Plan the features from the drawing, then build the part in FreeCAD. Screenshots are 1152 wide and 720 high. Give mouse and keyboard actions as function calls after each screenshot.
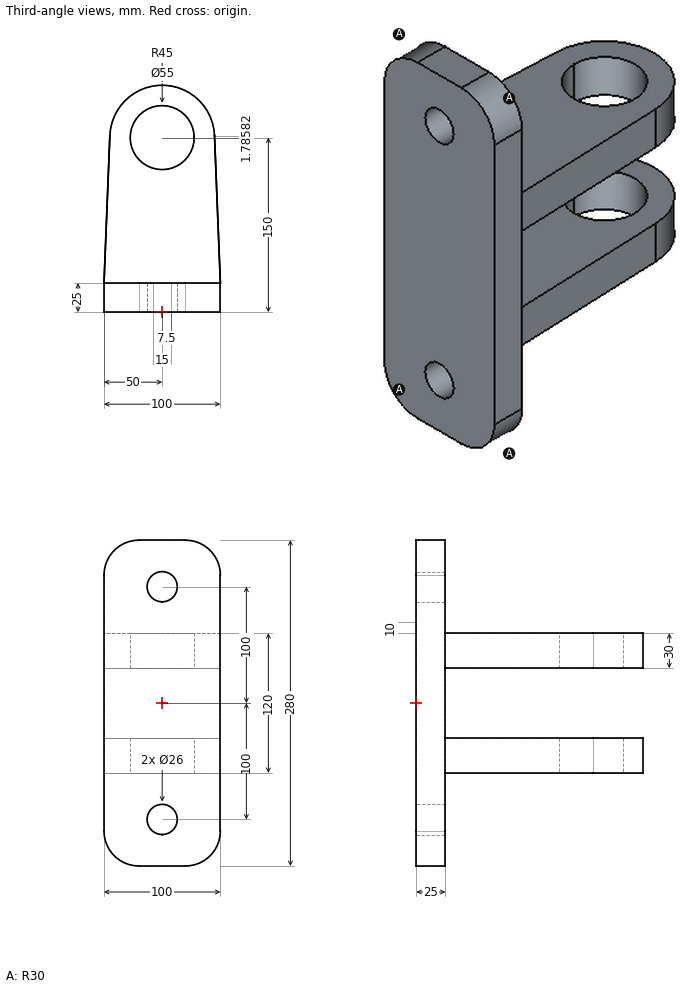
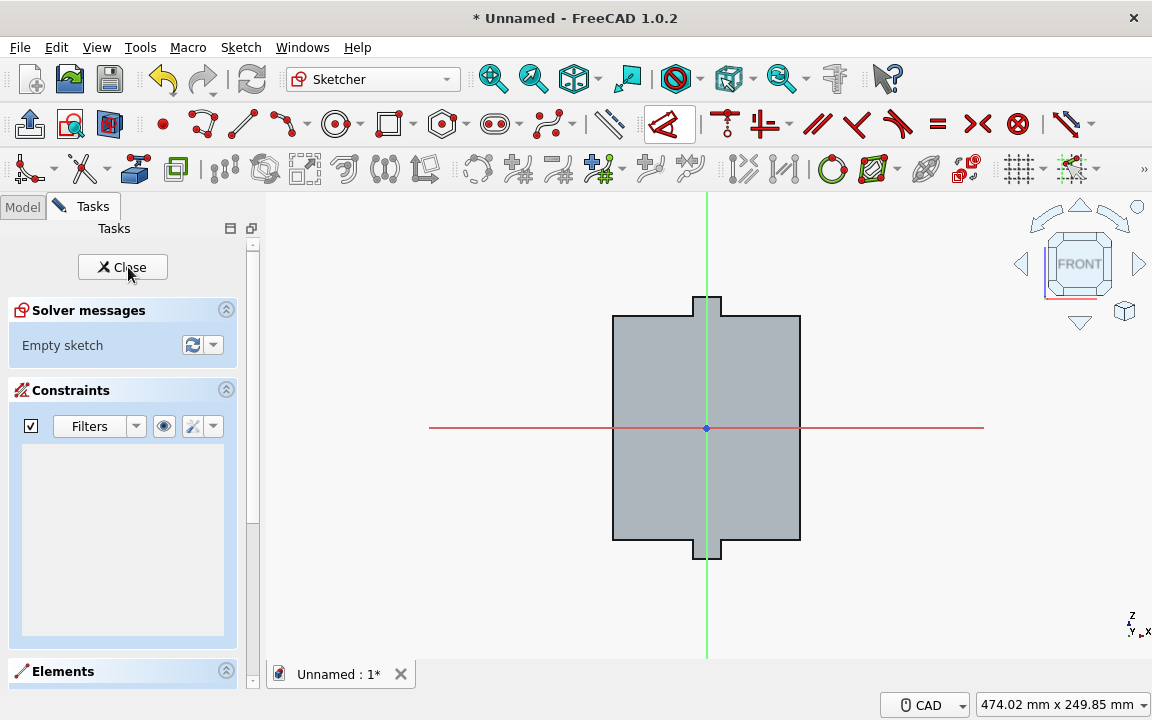
scroll(560, 422, down, 3)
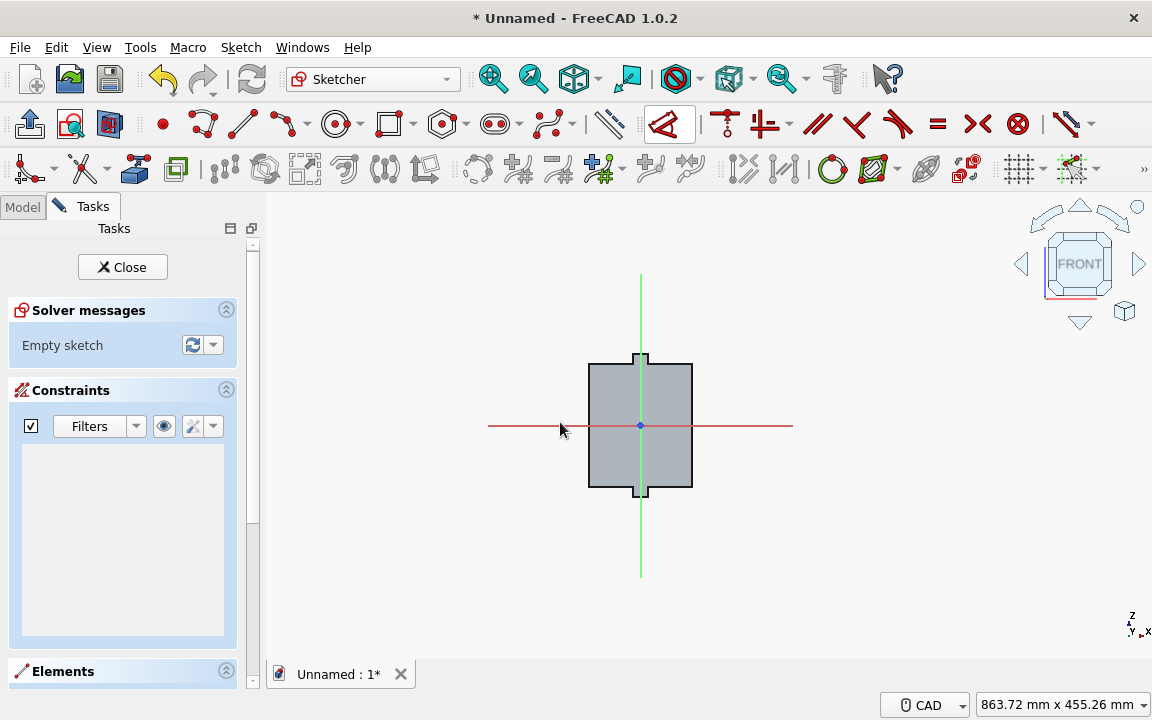
key(g)
key(v)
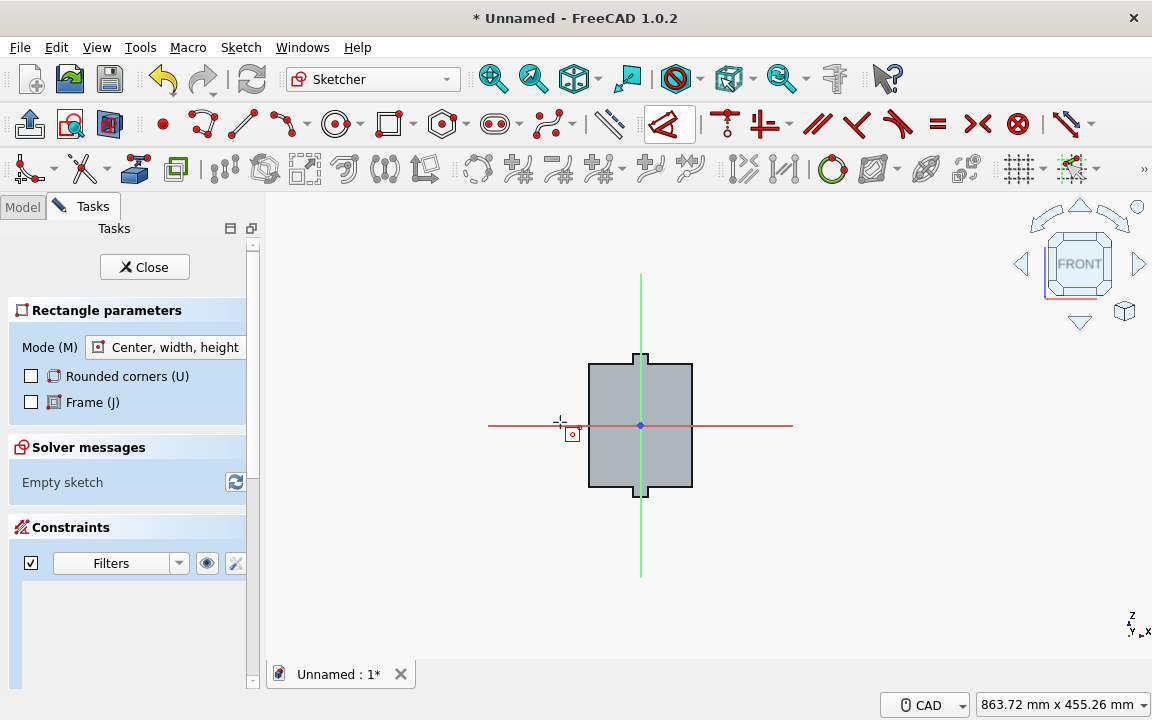
click(641, 426)
click(692, 282)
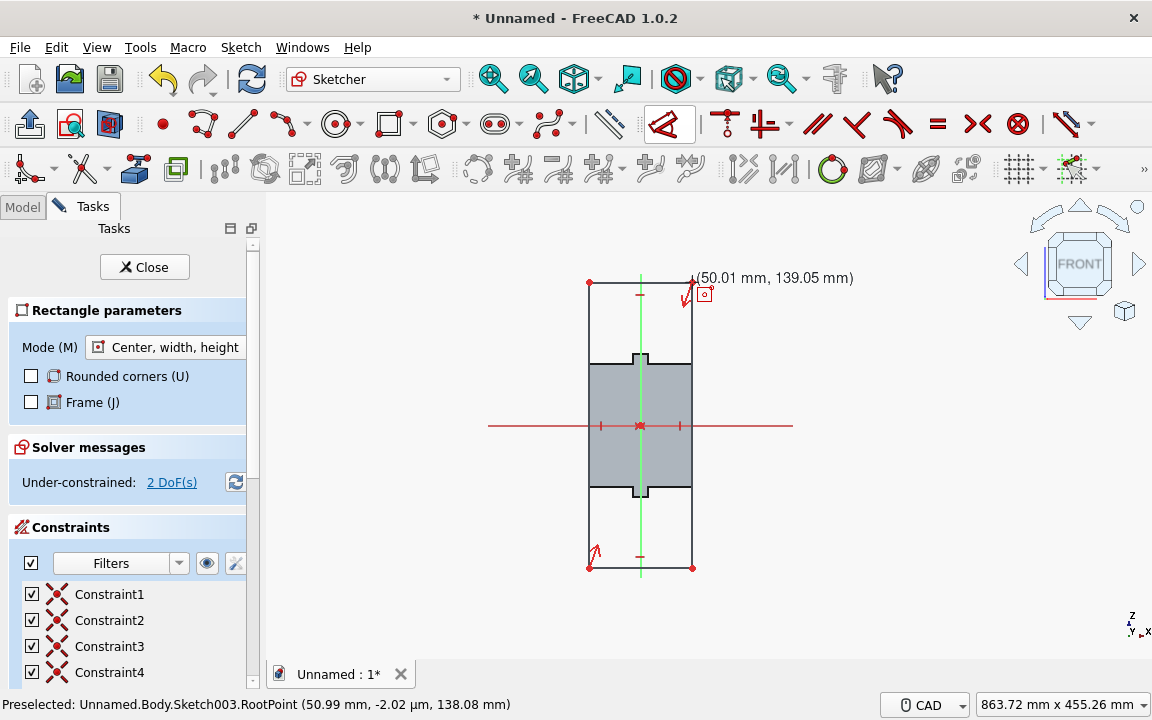
click(336, 124)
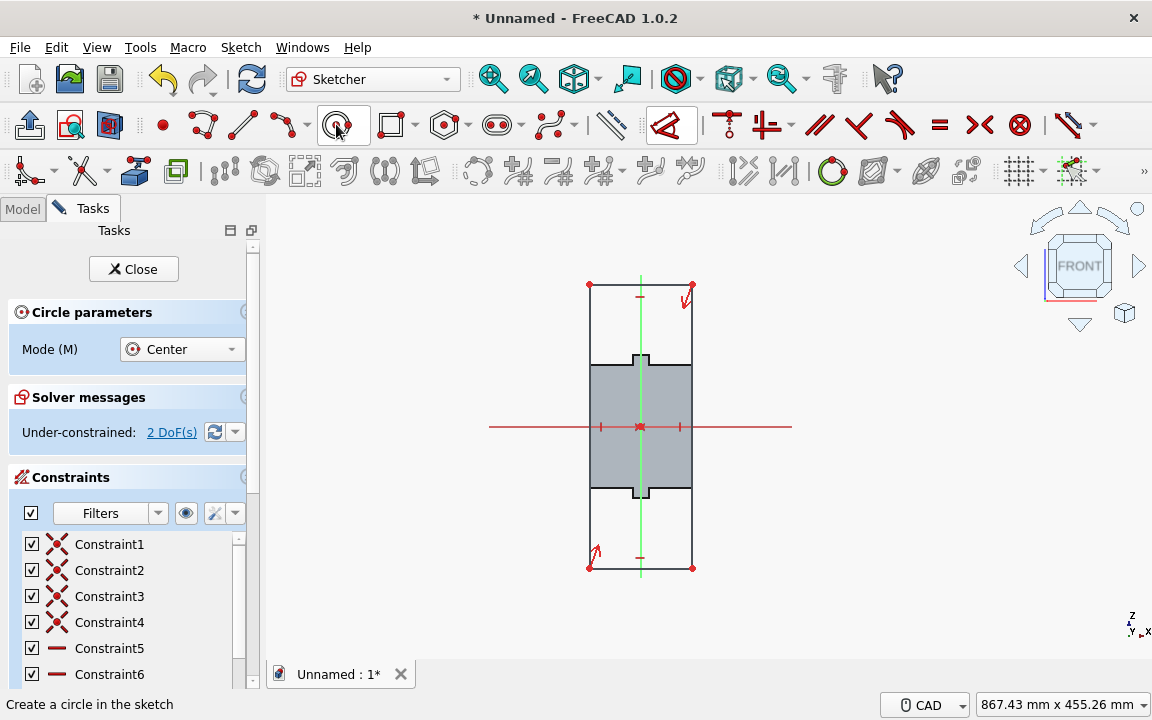
scroll(641, 529, up, 3)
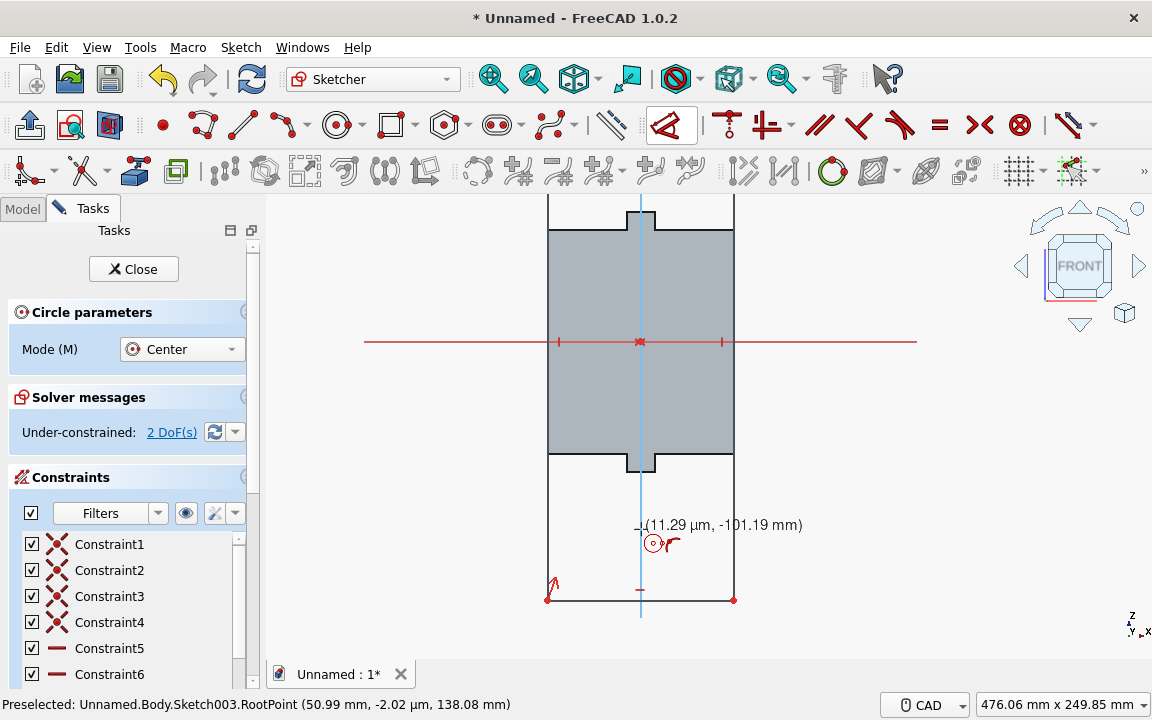
click(641, 528)
click(658, 511)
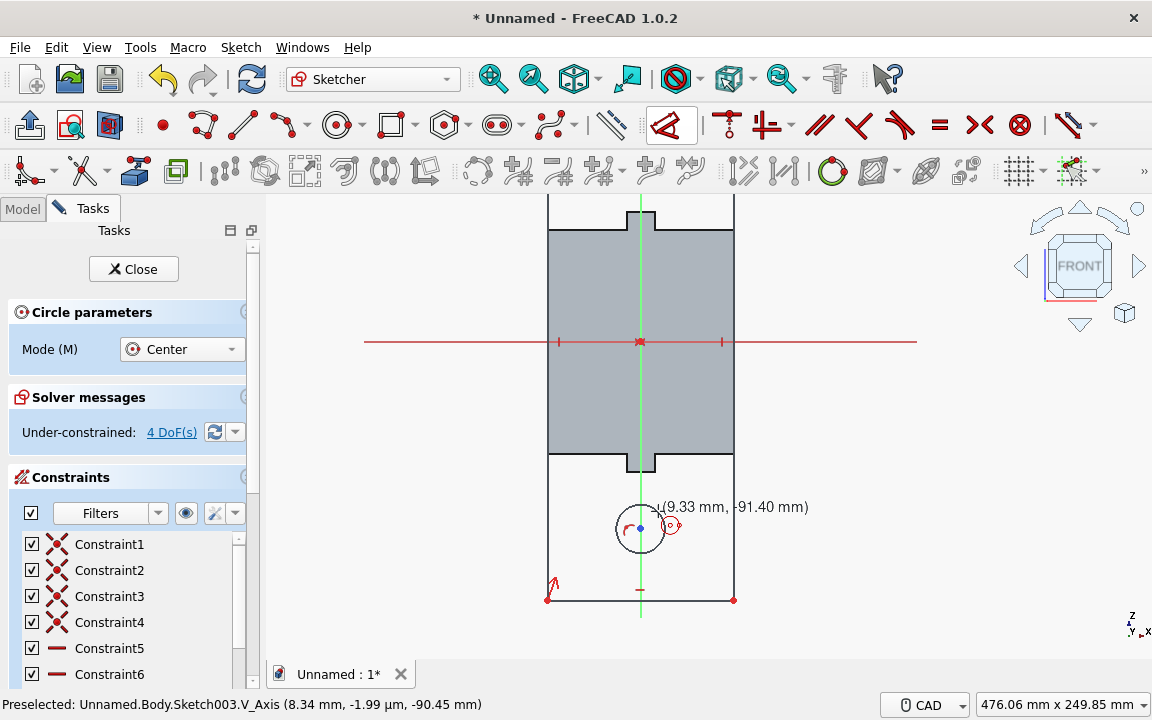
scroll(640, 529, down, 3)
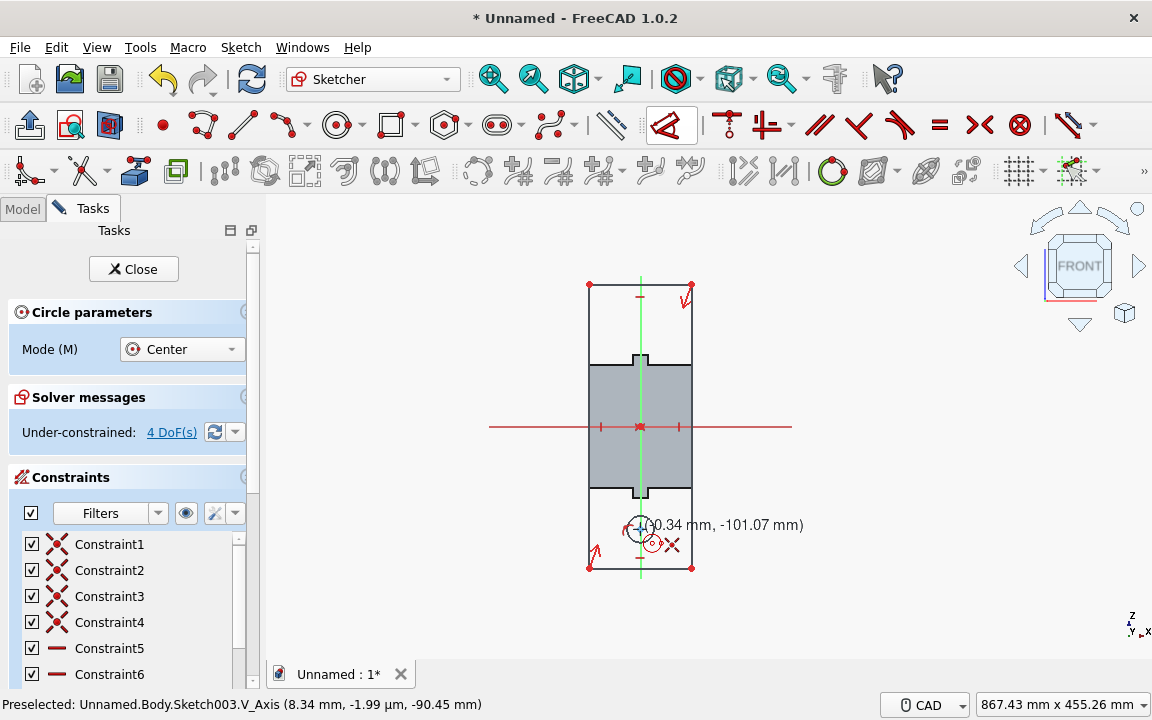
scroll(641, 324, up, 3)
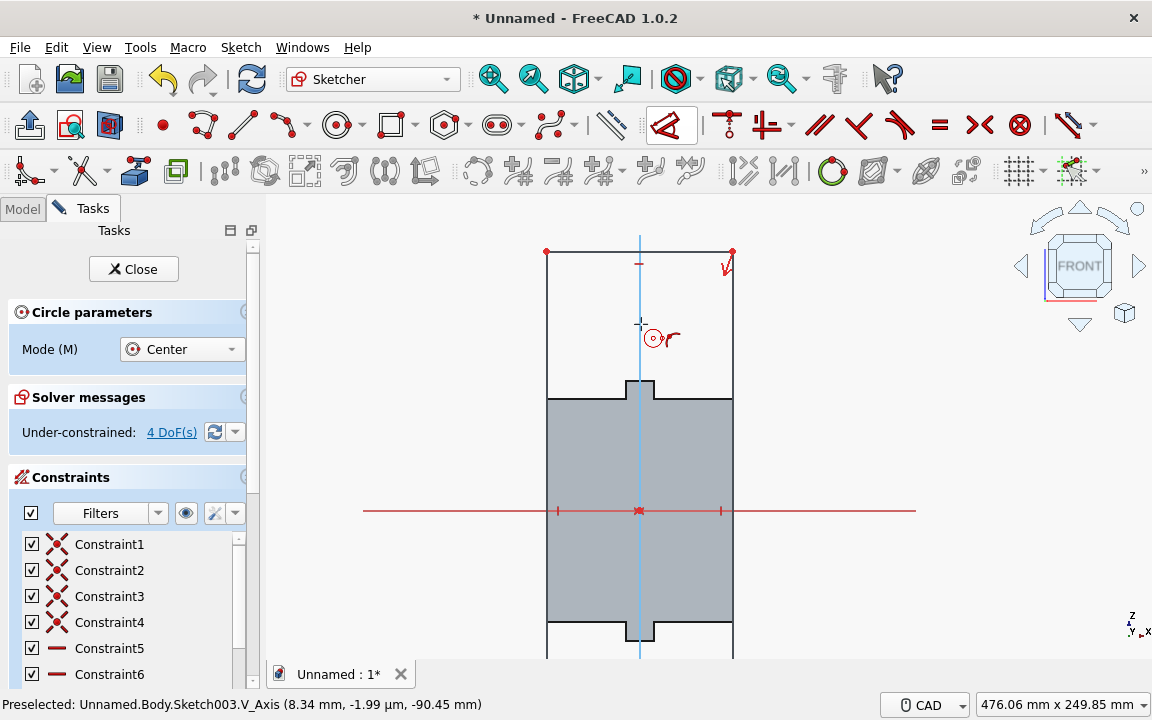
click(640, 325)
click(657, 308)
key(Escape)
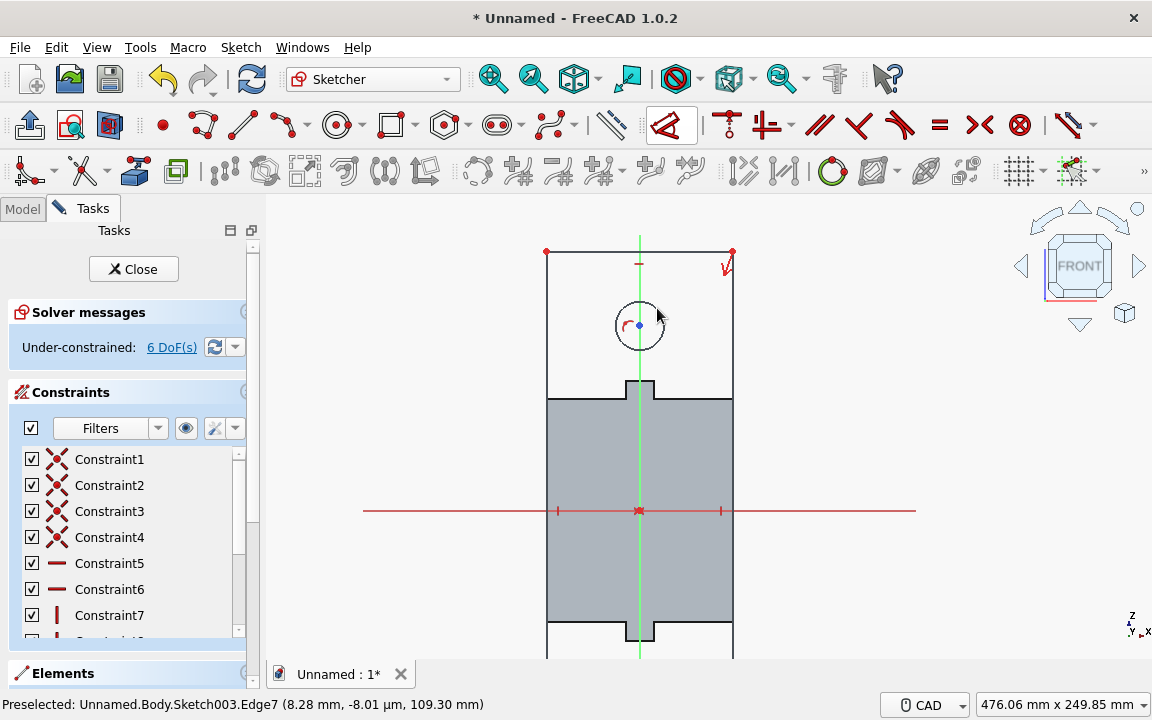
scroll(641, 324, down, 3)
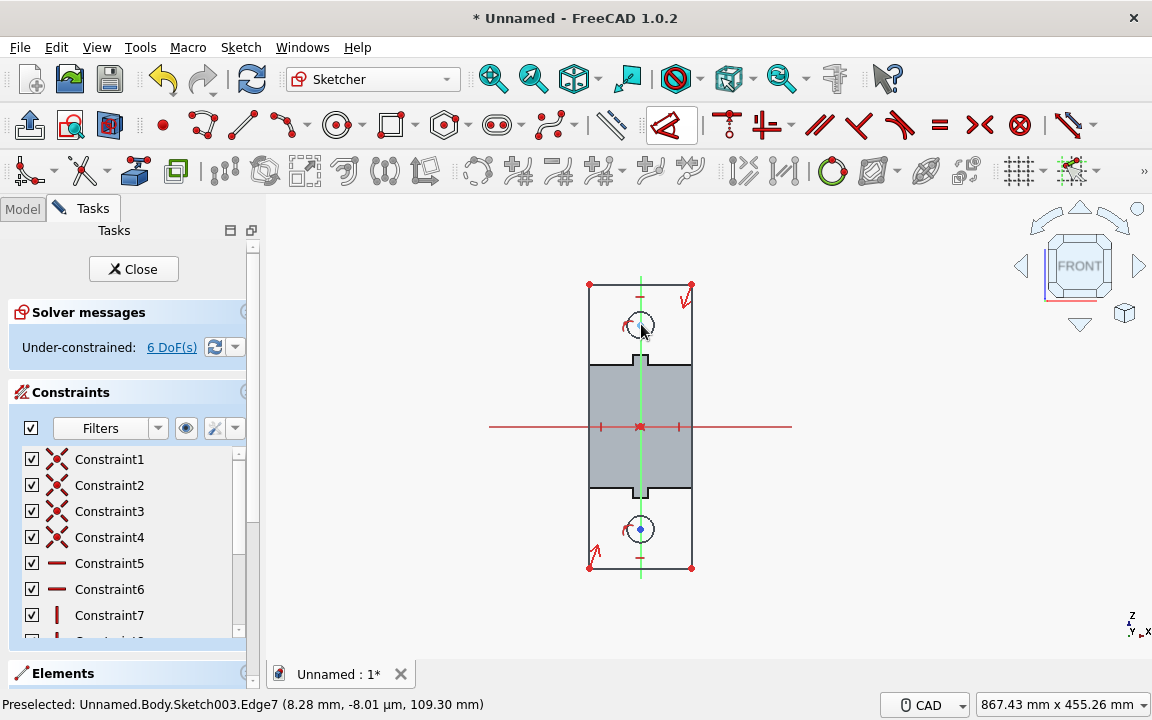
scroll(650, 520, up, 2)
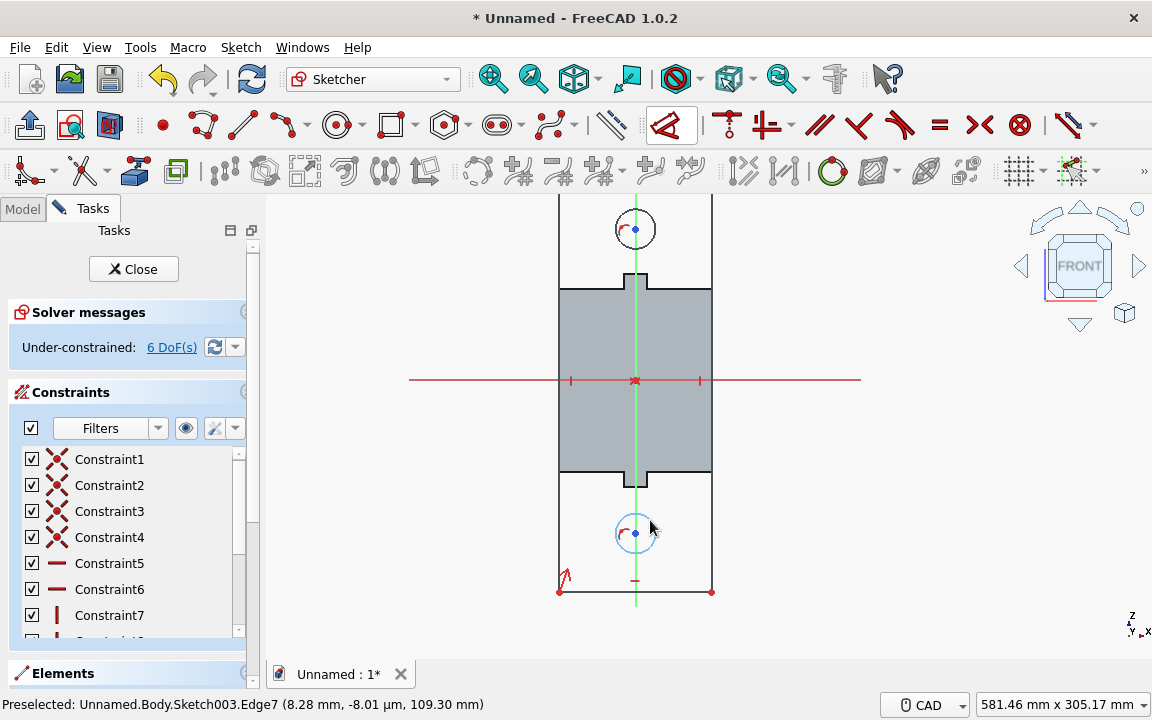
click(650, 519)